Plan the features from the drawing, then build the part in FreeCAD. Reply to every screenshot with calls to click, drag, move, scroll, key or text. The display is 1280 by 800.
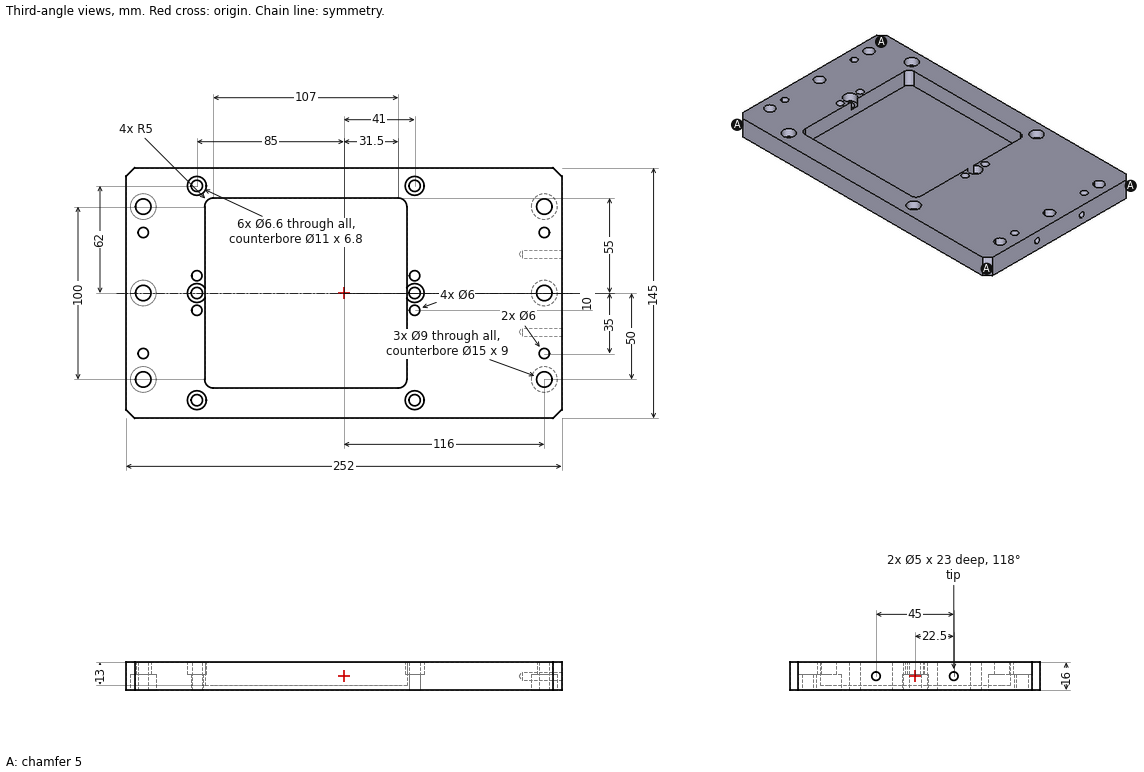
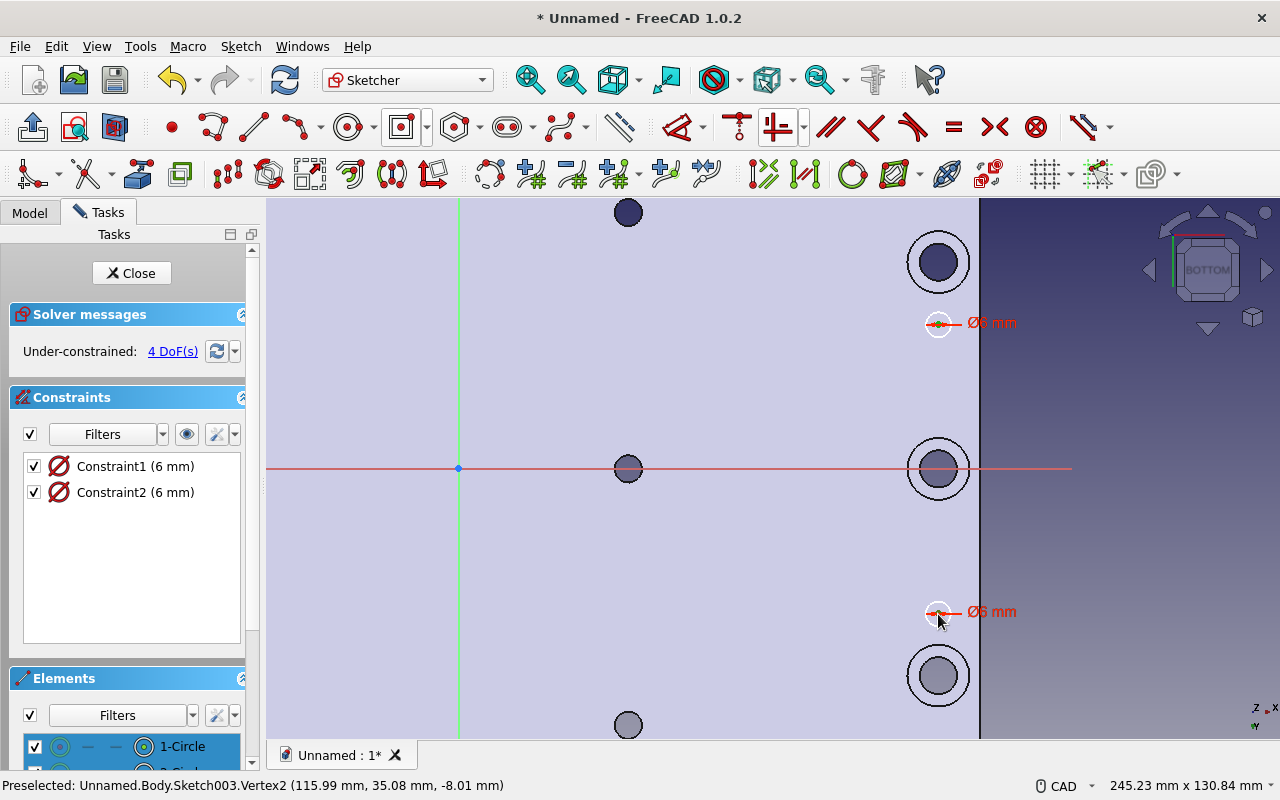
click(353, 469)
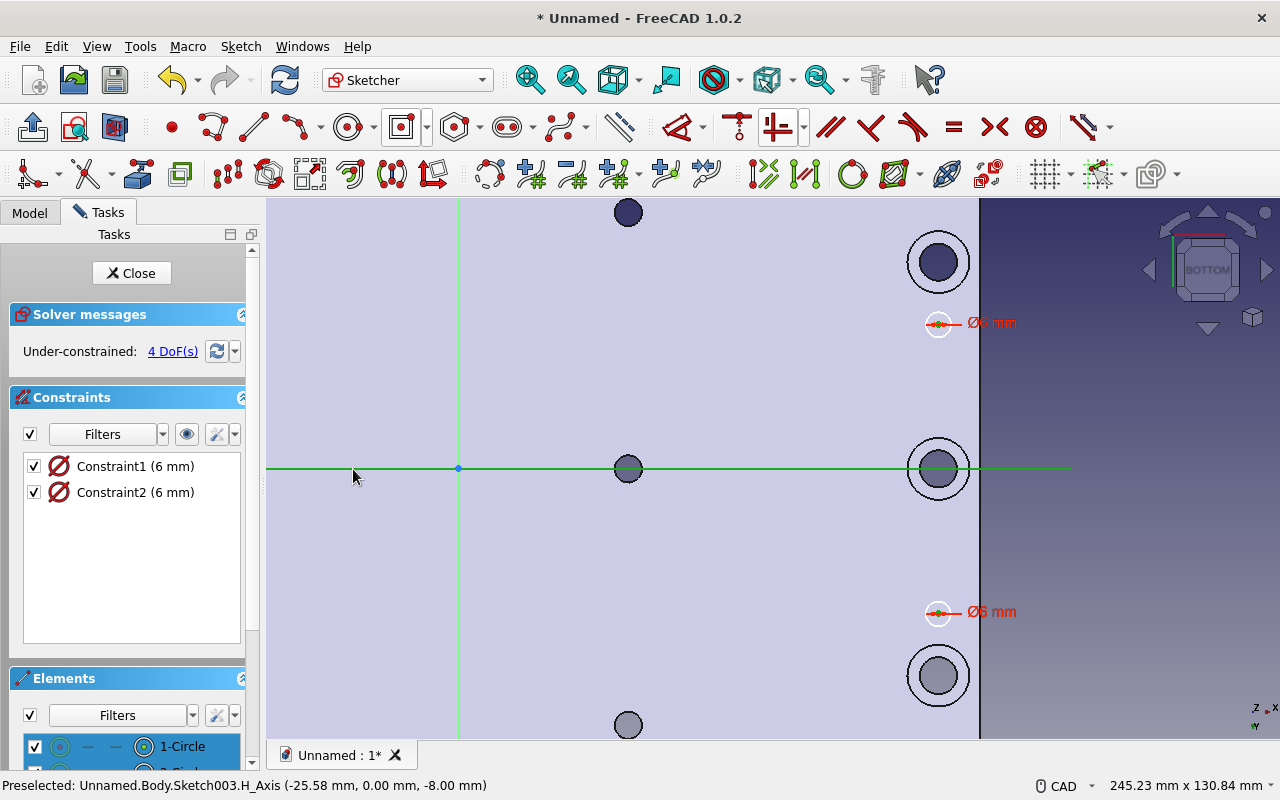
click(995, 128)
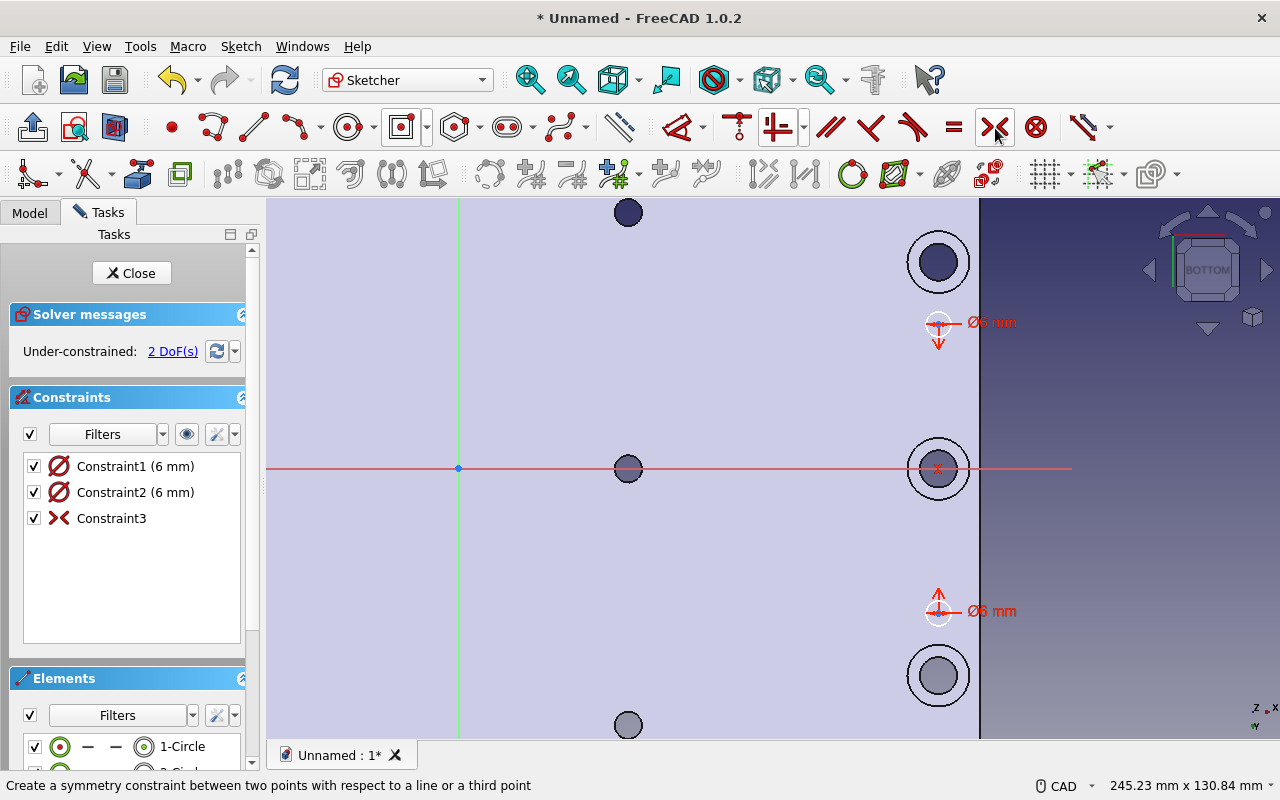
click(676, 128)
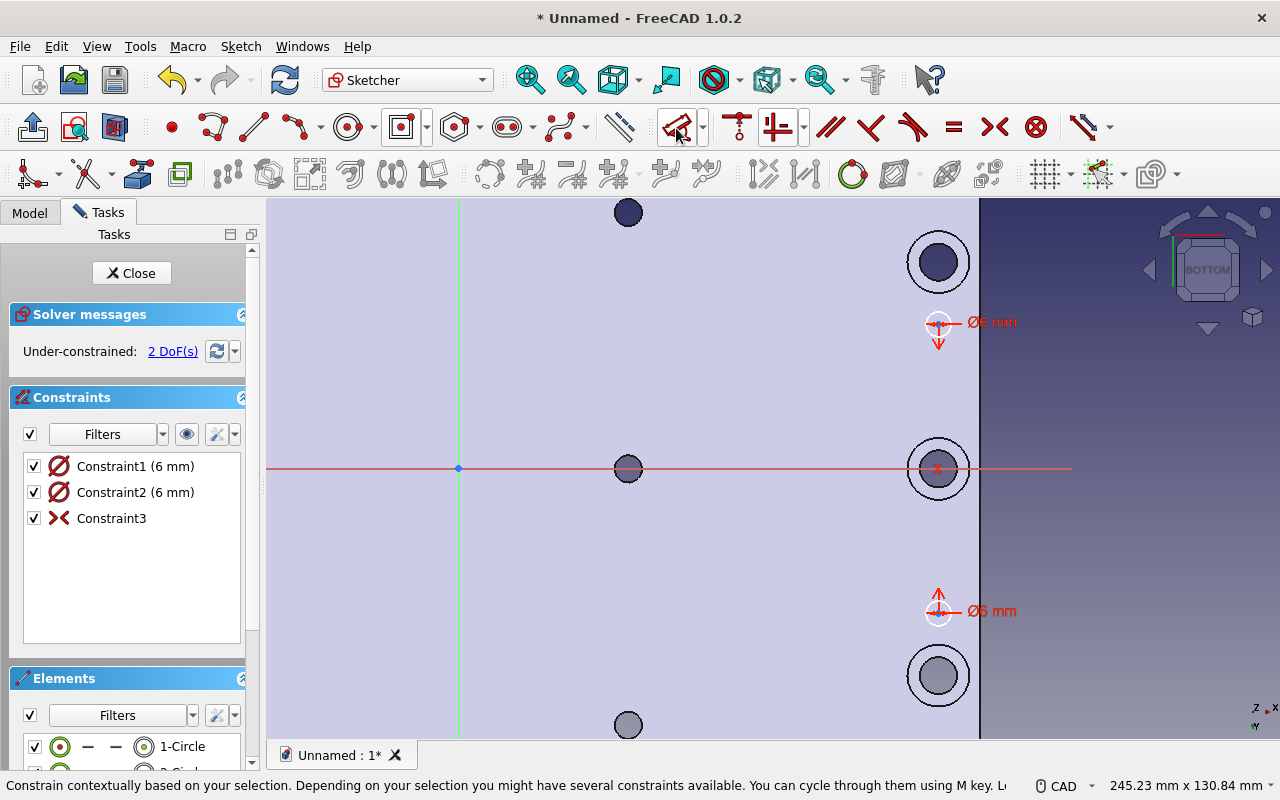
click(939, 324)
click(425, 397)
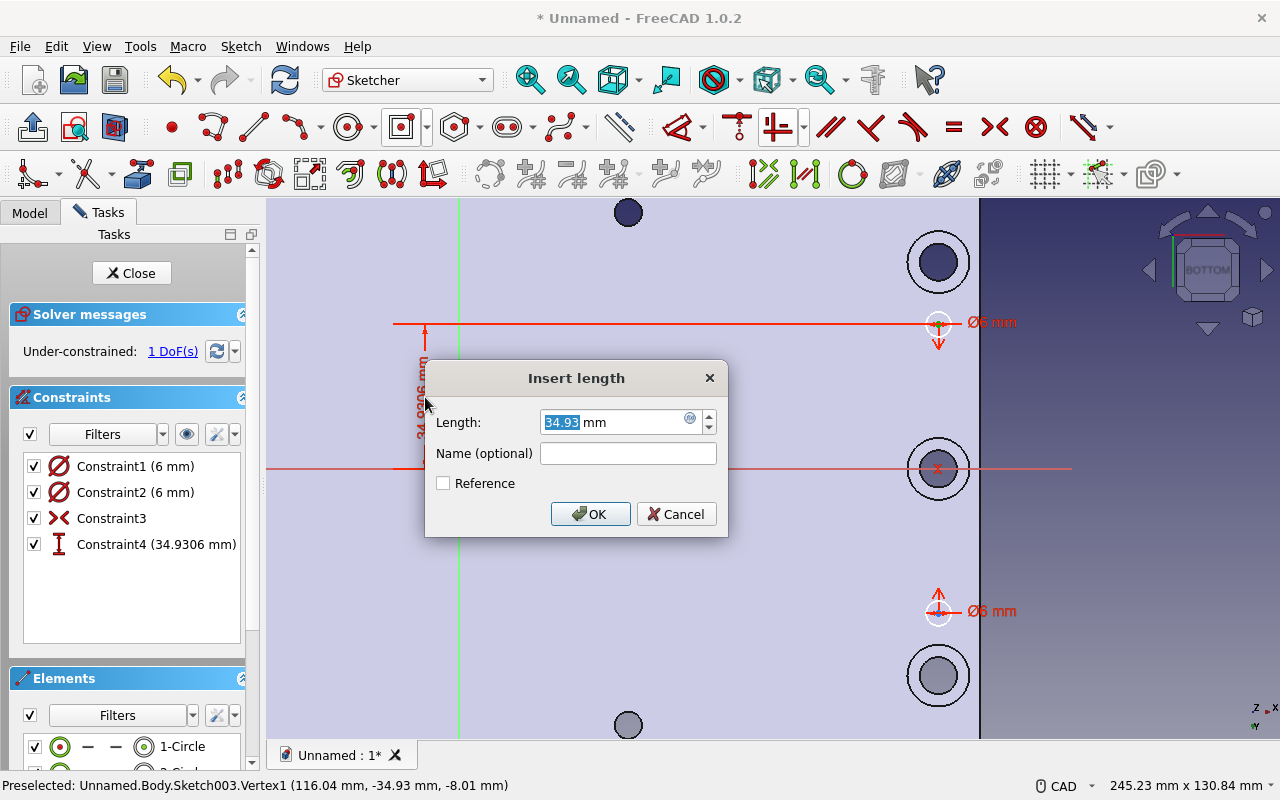
text(35)
key(Return)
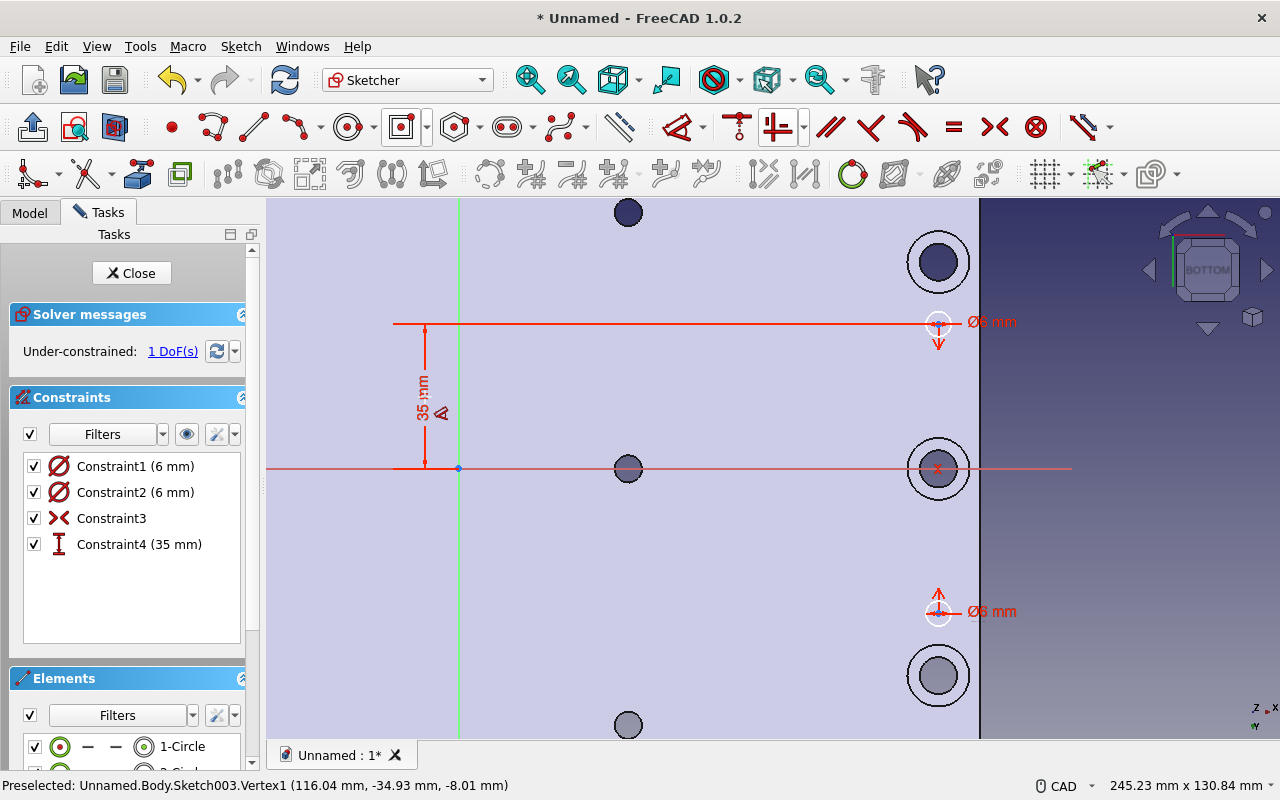
click(939, 324)
click(699, 290)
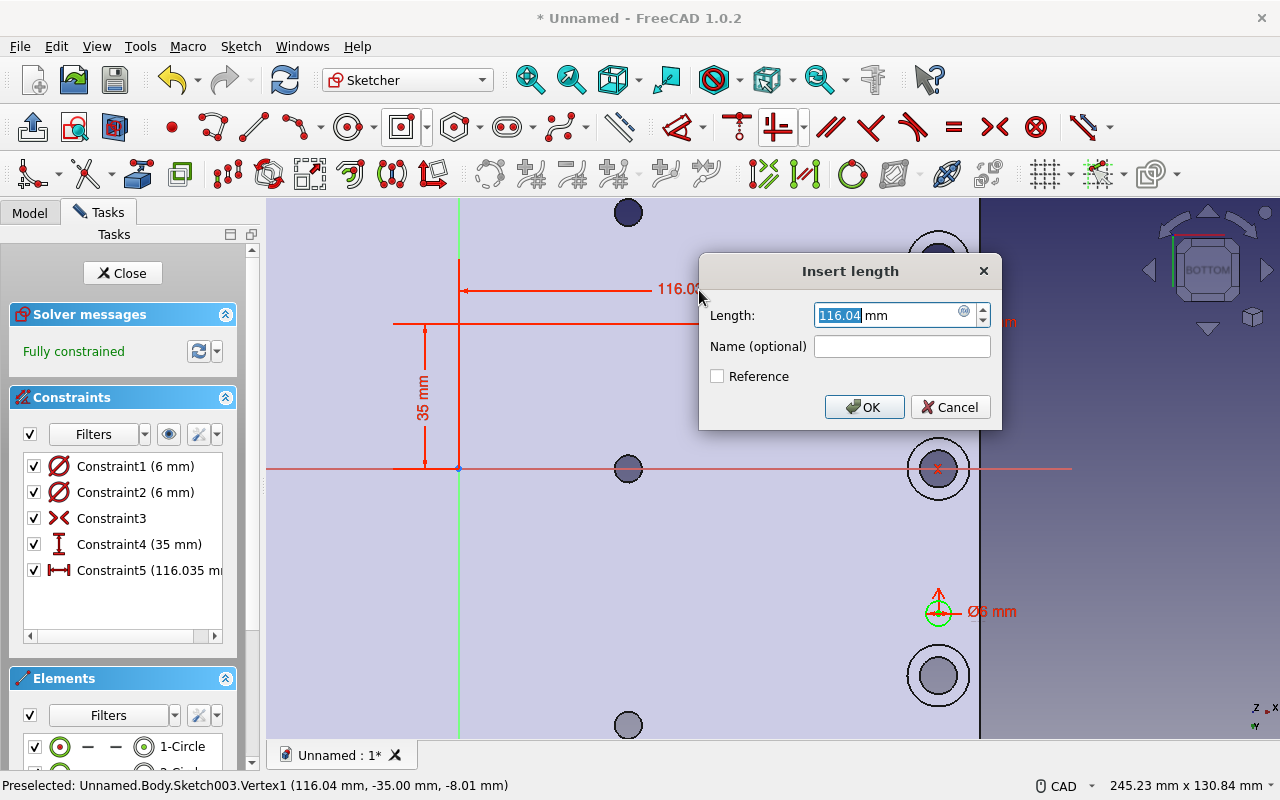
text(116)
key(Return)
key(Escape)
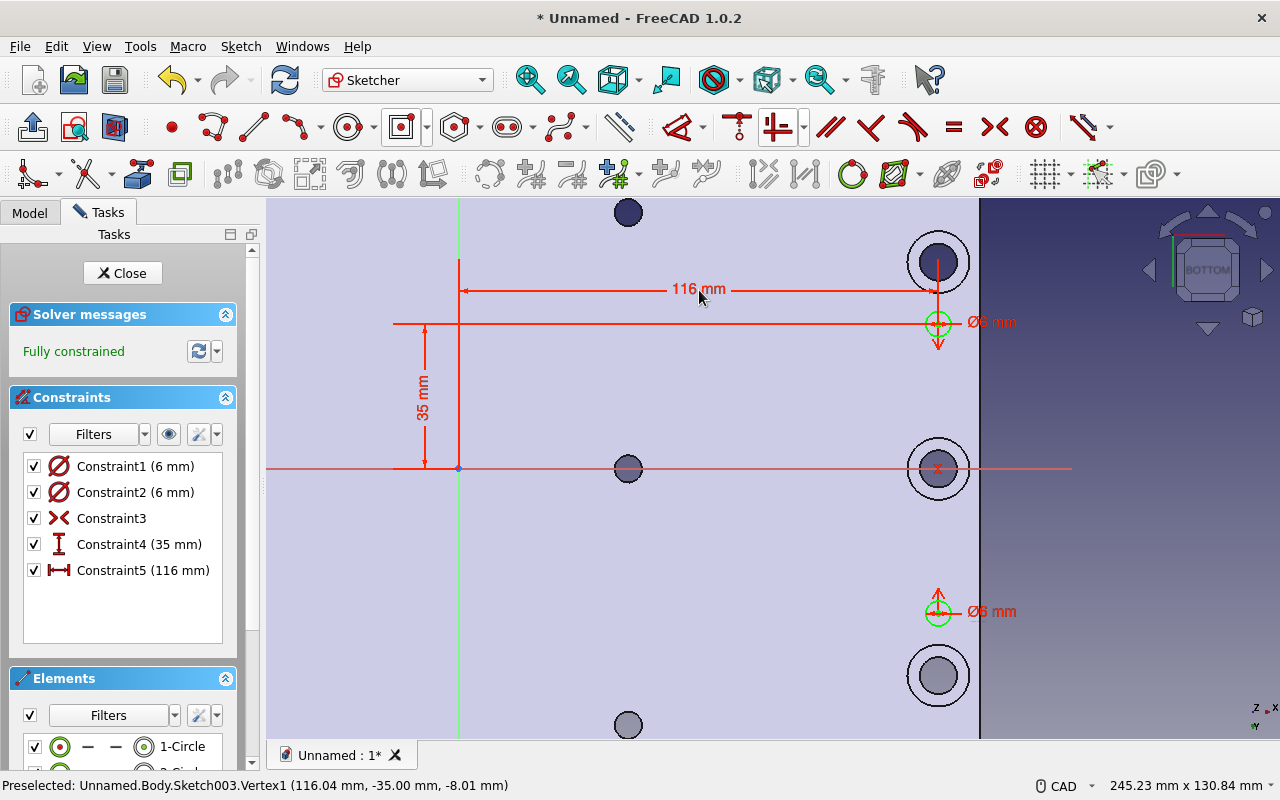
click(123, 273)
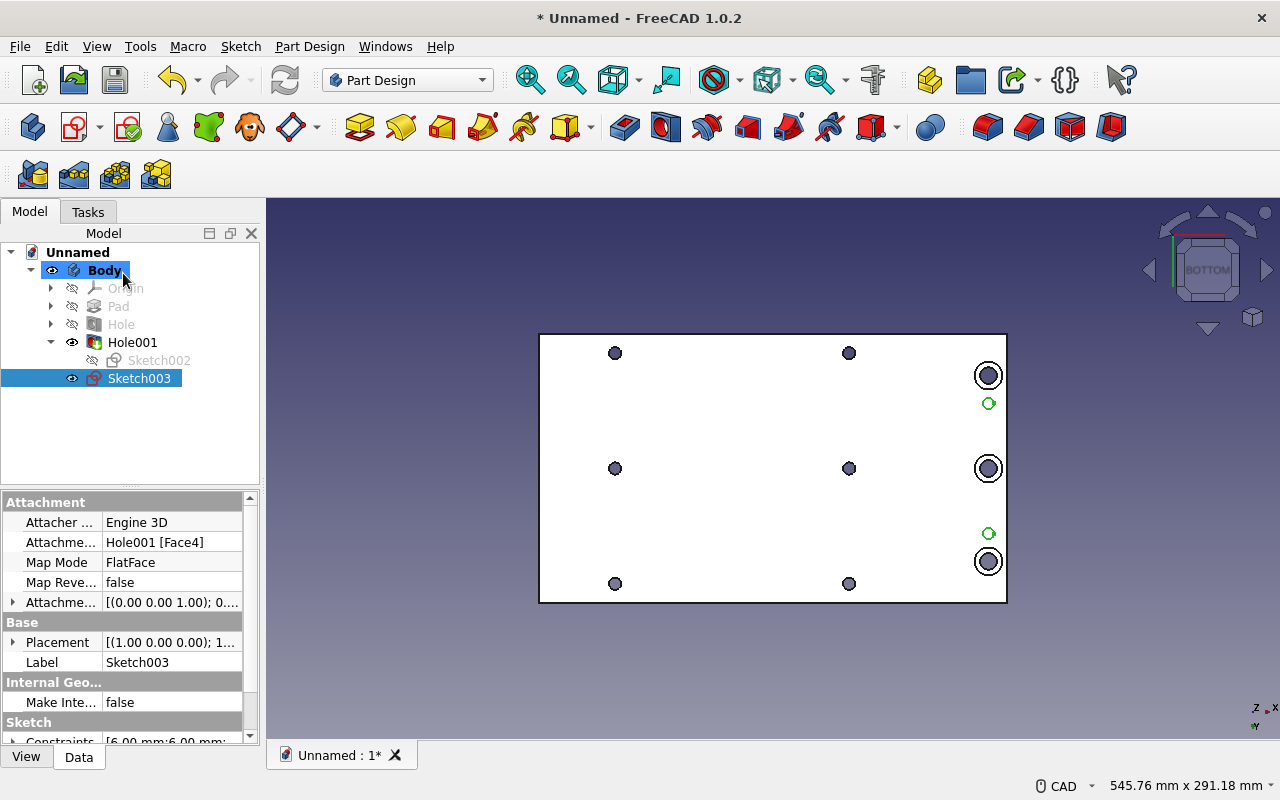
click(625, 128)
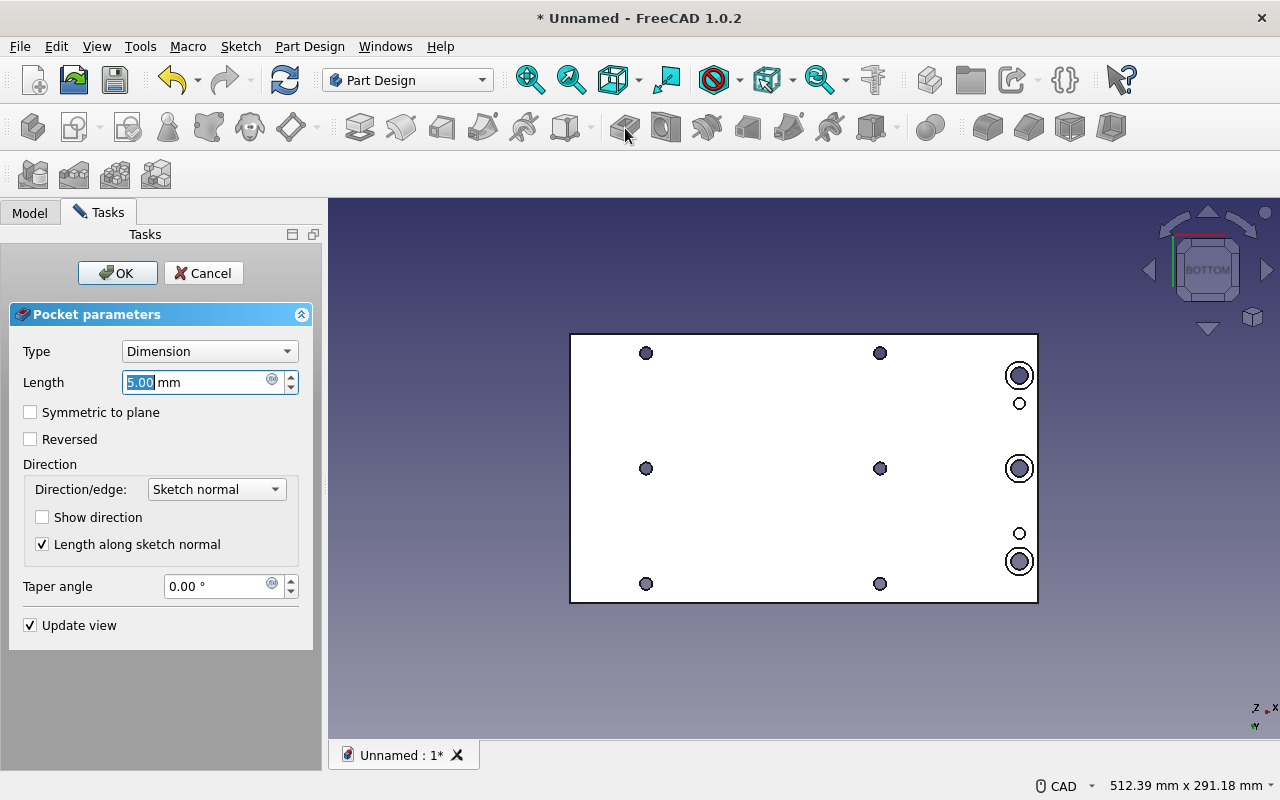
click(210, 352)